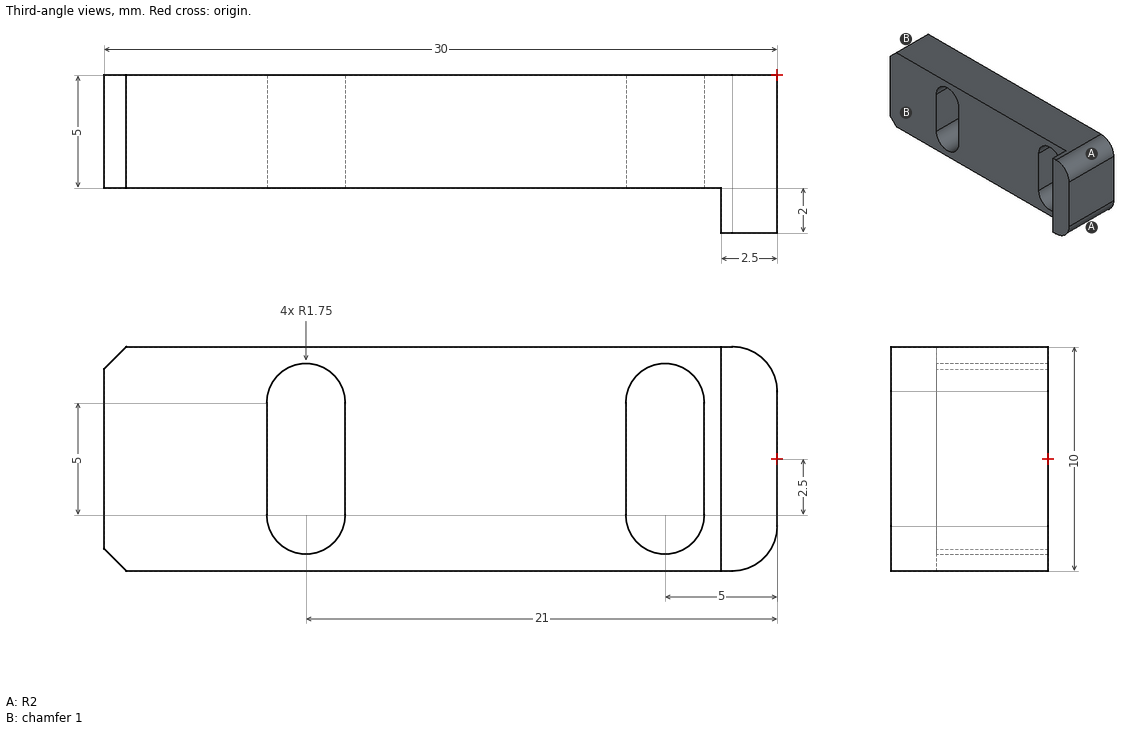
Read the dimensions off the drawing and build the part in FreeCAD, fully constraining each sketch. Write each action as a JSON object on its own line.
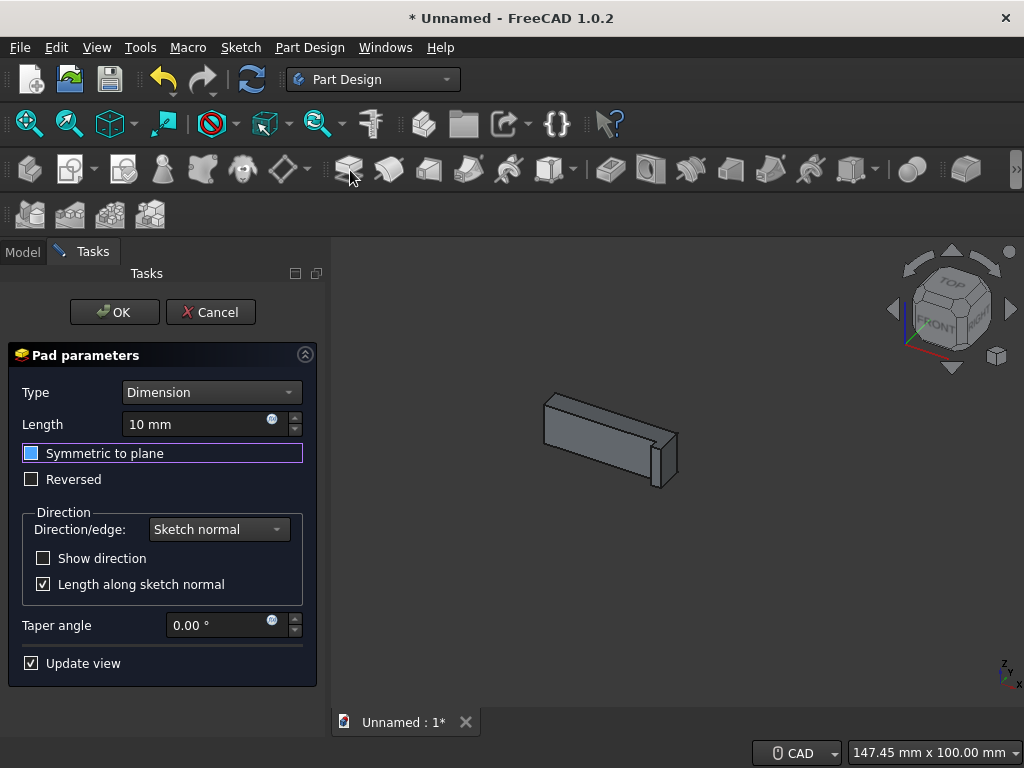
{"action": "left_click", "coordinate": [30, 453]}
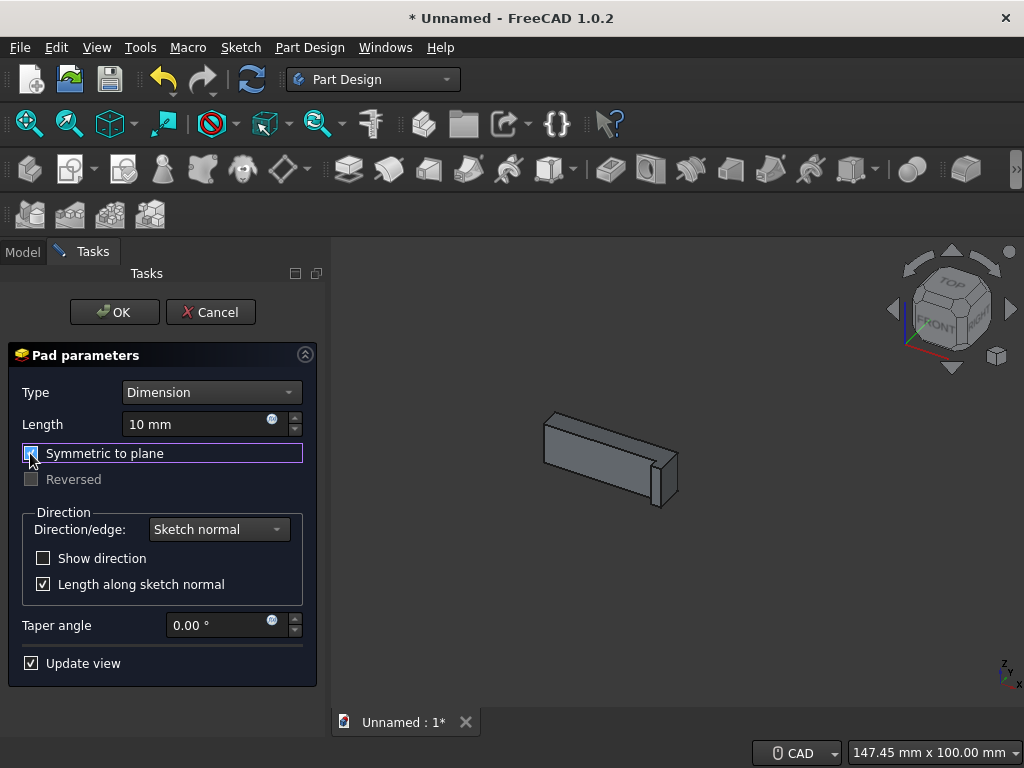
{"action": "left_click", "coordinate": [115, 312]}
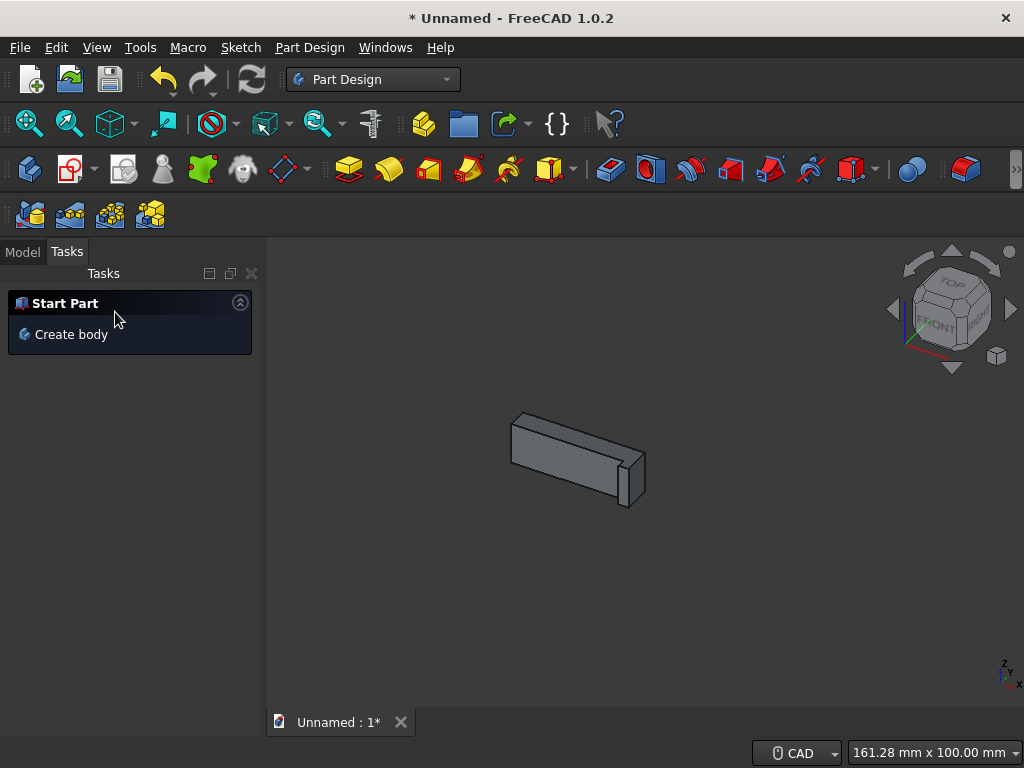
{"action": "key", "text": "v f"}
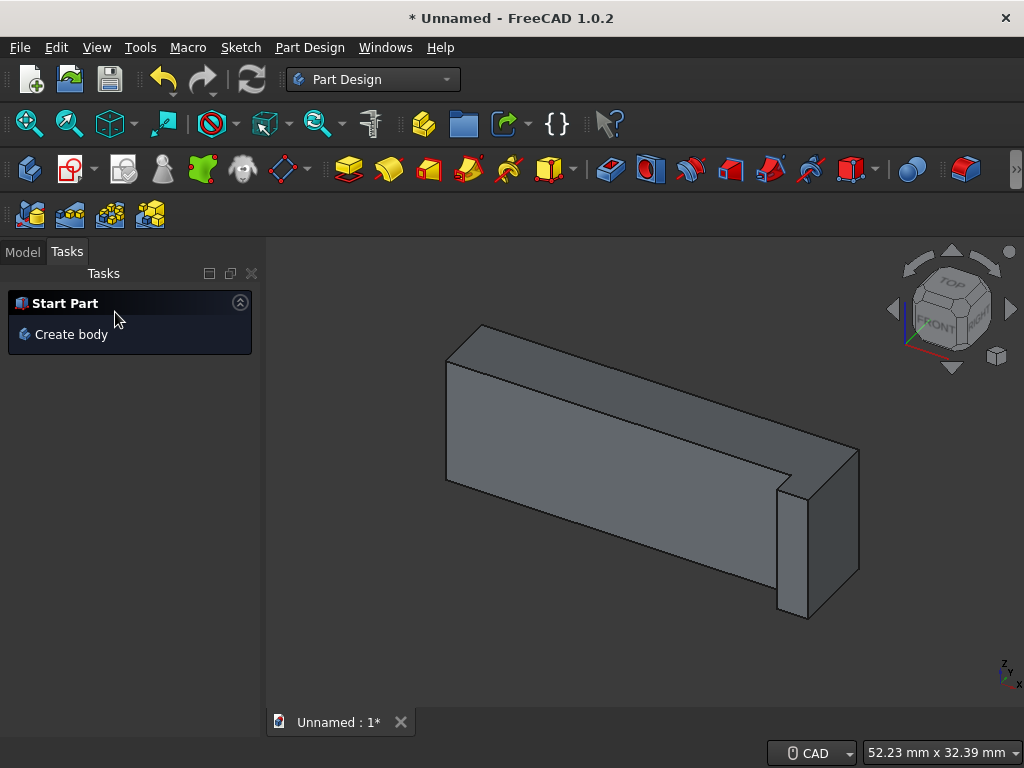
{"action": "left_click", "coordinate": [717, 509]}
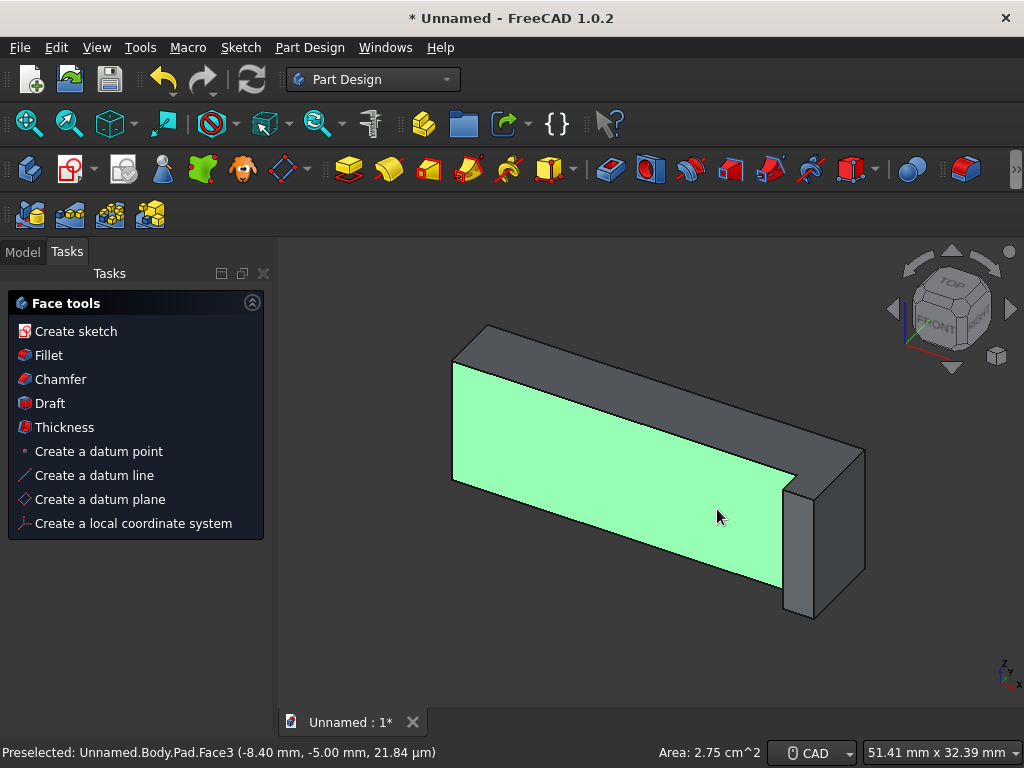
{"action": "left_click", "coordinate": [70, 170]}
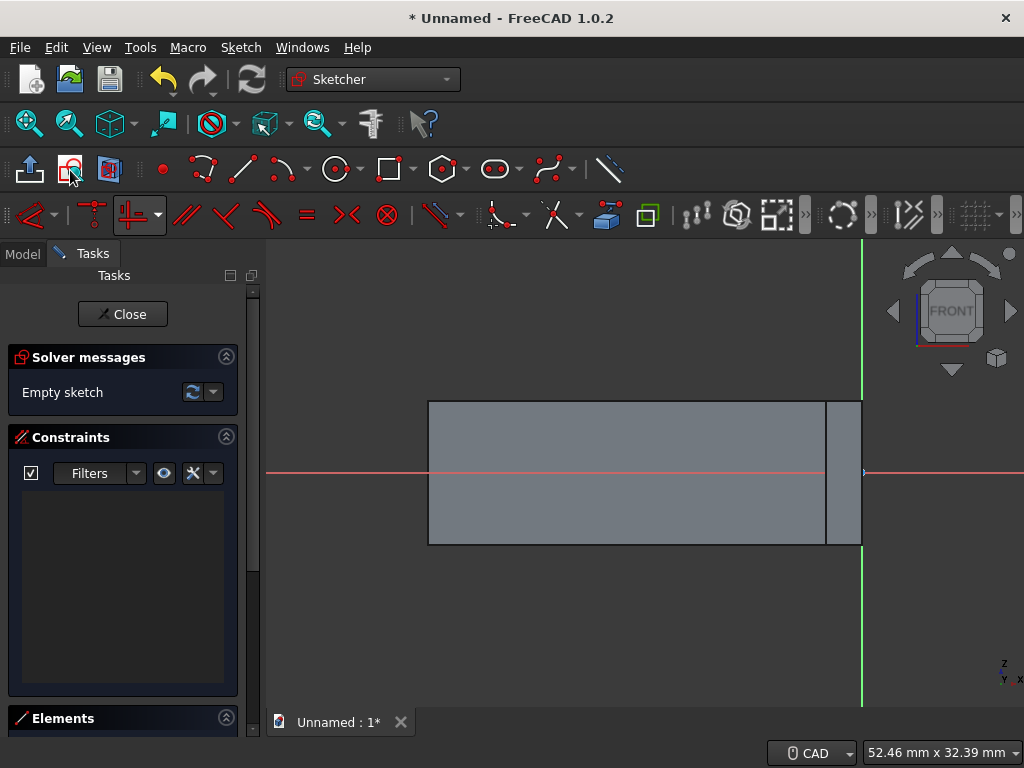
{"action": "scroll", "coordinate": [294, 473], "scroll_direction": "down", "scroll_amount": 1}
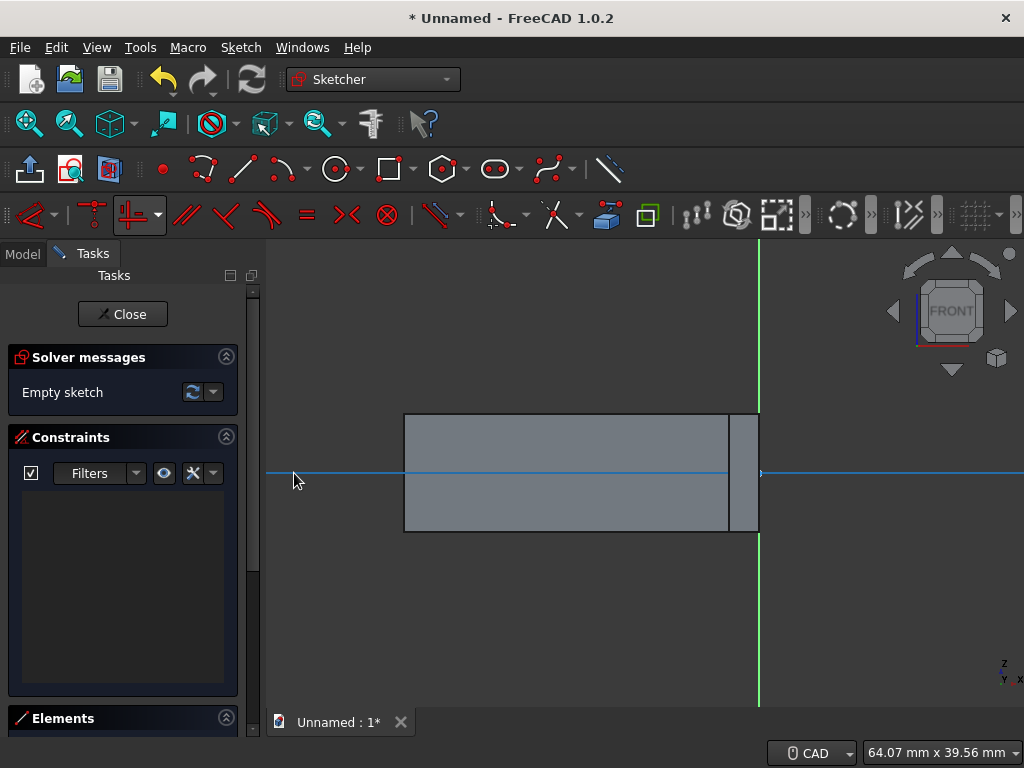
{"action": "scroll", "coordinate": [721, 473], "scroll_direction": "up", "scroll_amount": 2}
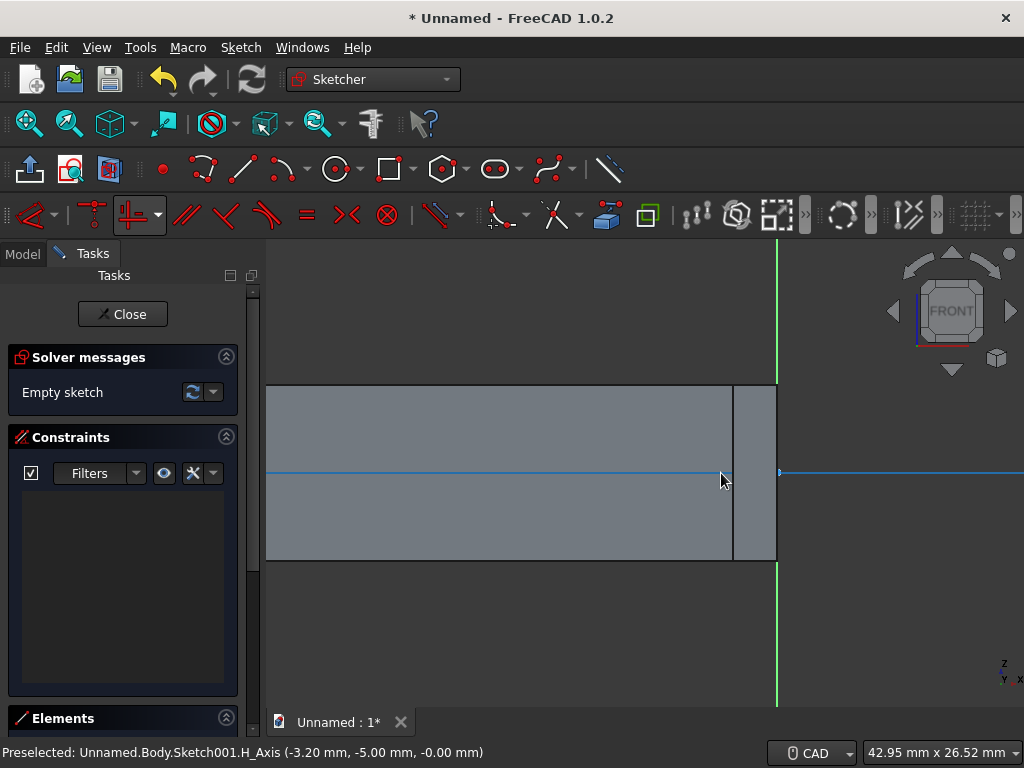
{"action": "left_click", "coordinate": [496, 170]}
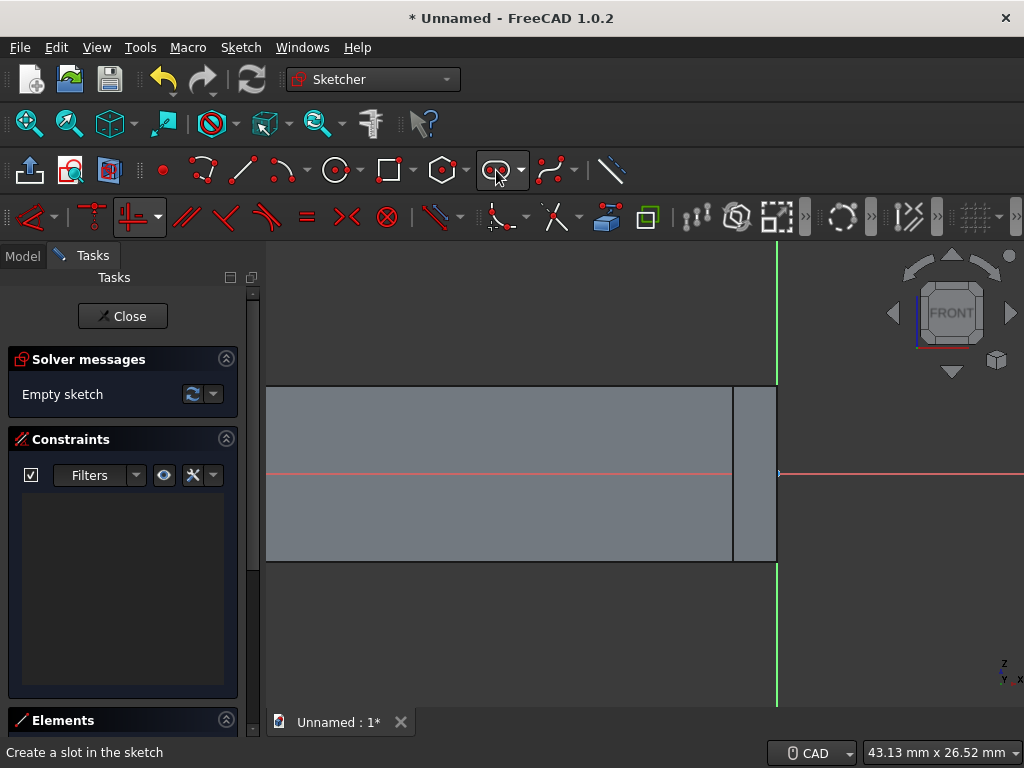
{"action": "left_click", "coordinate": [408, 518]}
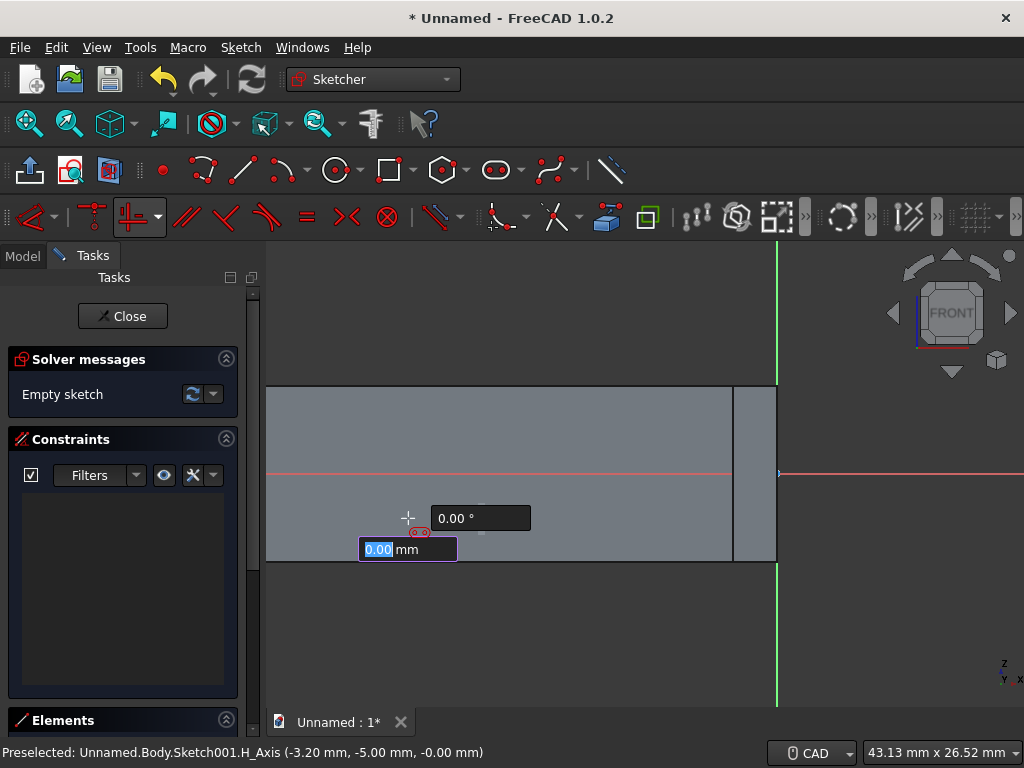
{"action": "left_click", "coordinate": [408, 430]}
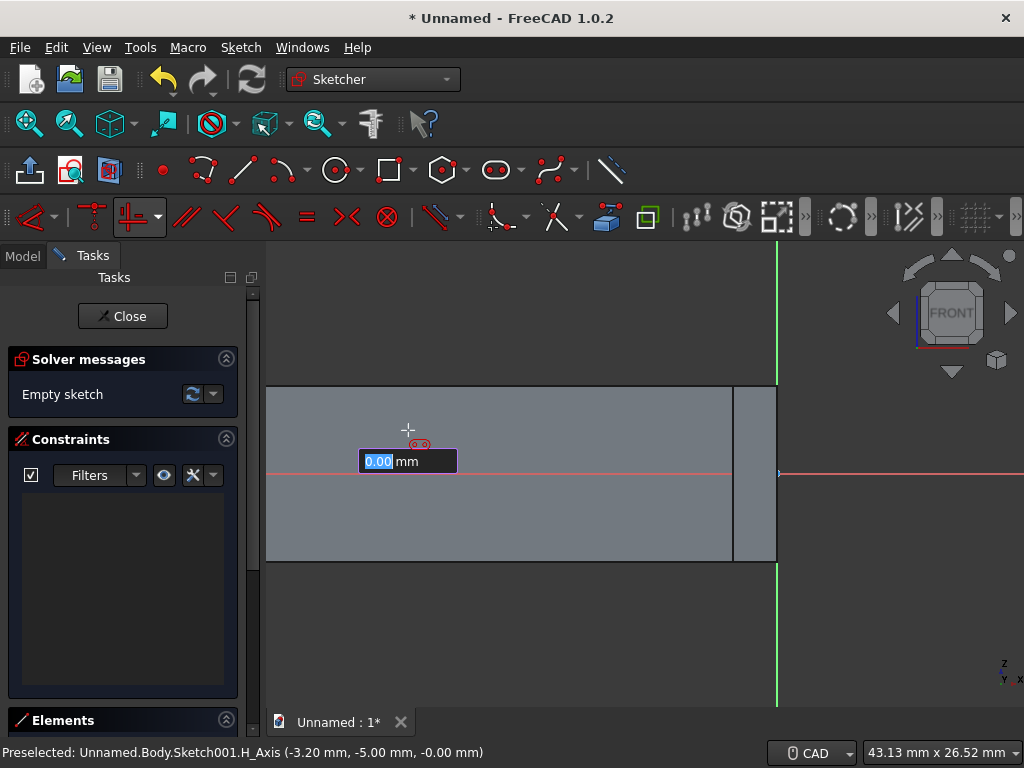
{"action": "left_click", "coordinate": [438, 487]}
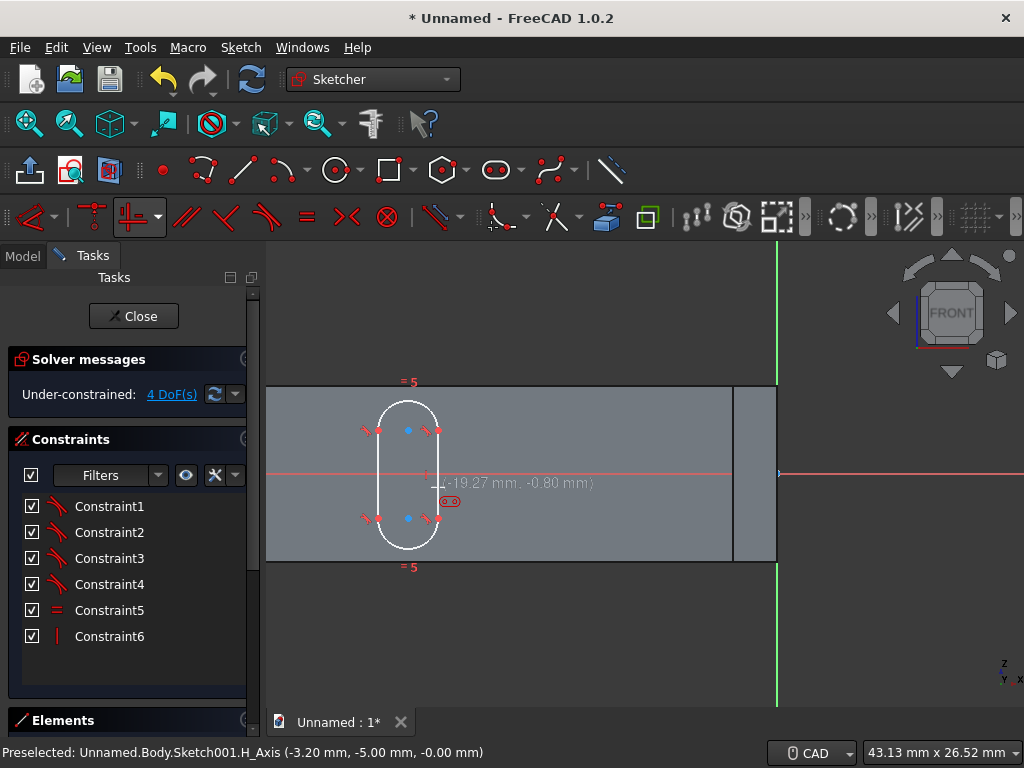
{"action": "left_click", "coordinate": [689, 518]}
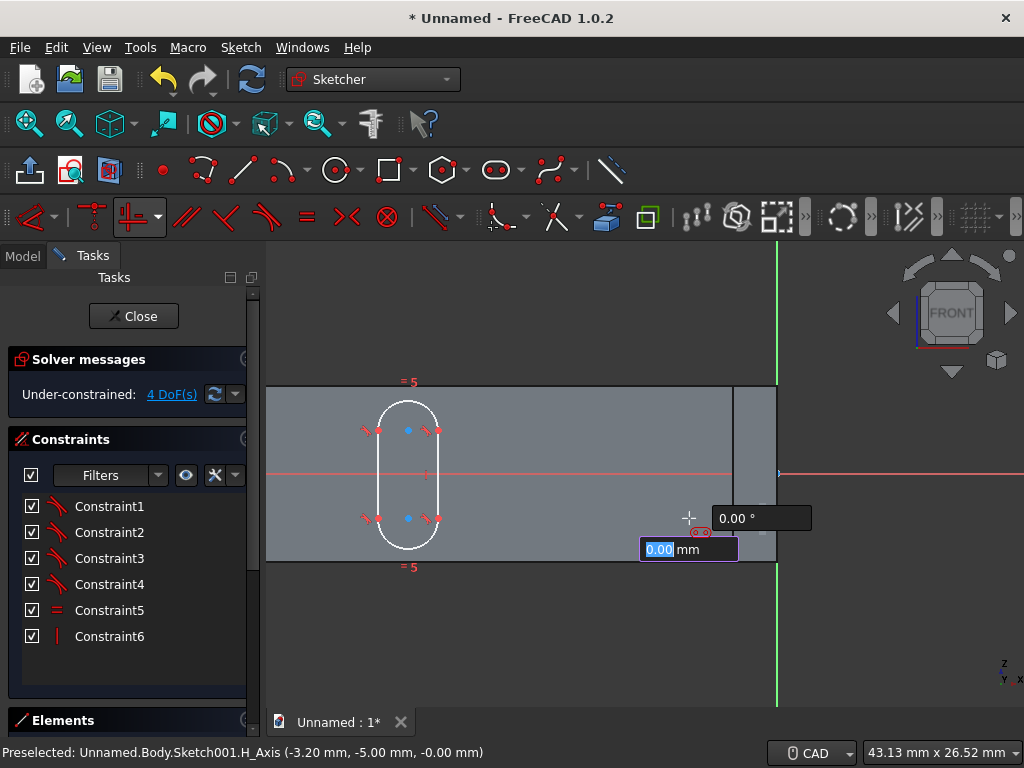
{"action": "left_click", "coordinate": [689, 430]}